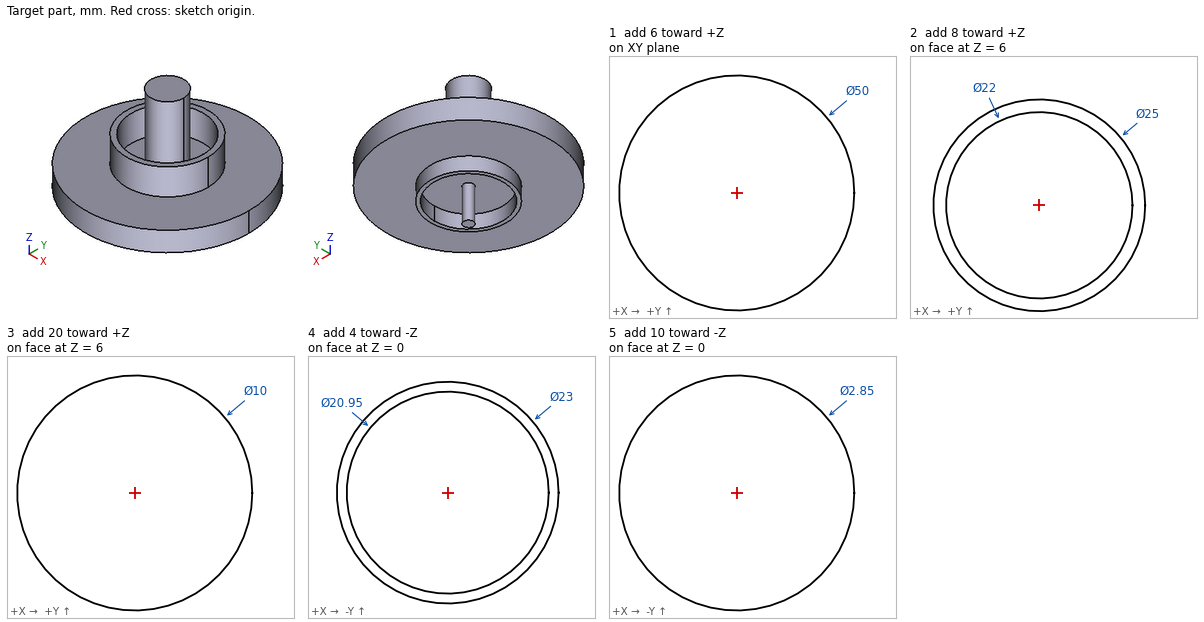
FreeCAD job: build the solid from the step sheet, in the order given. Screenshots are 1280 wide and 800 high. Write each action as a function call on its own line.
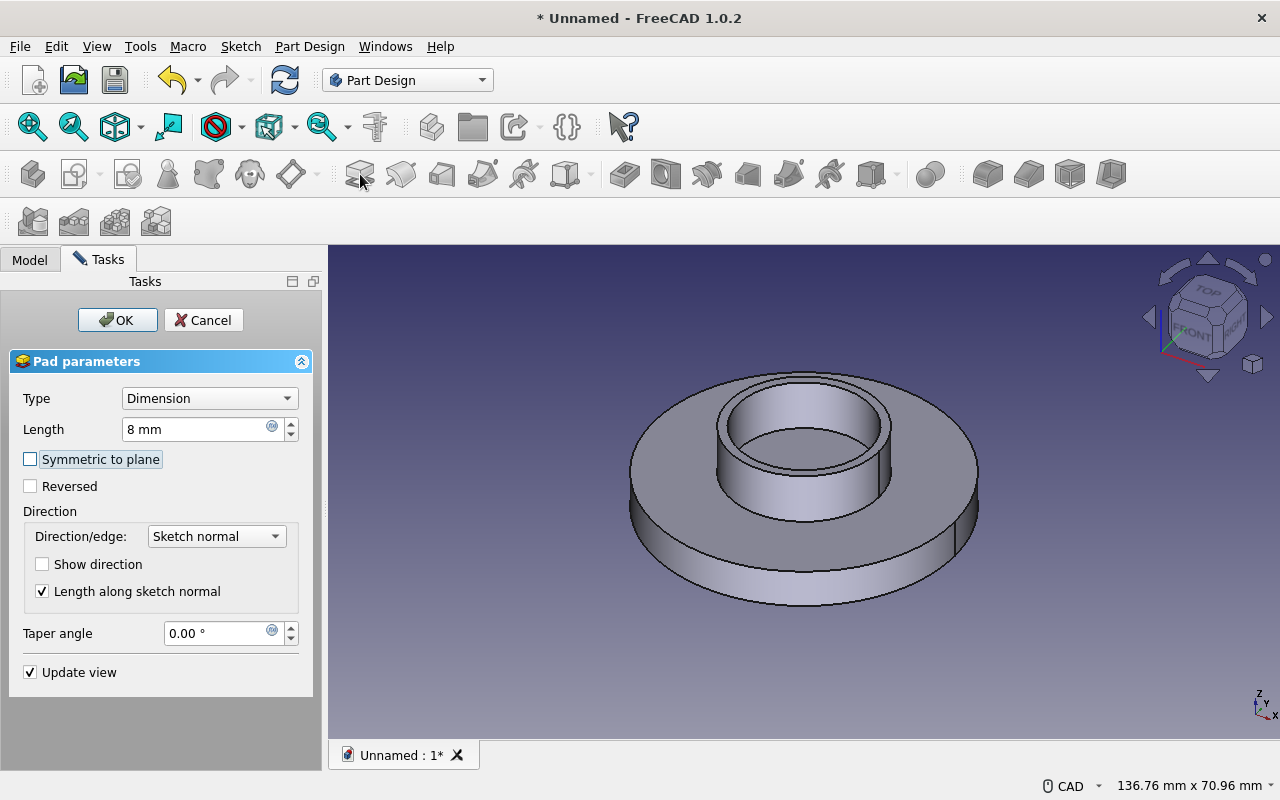
click(118, 320)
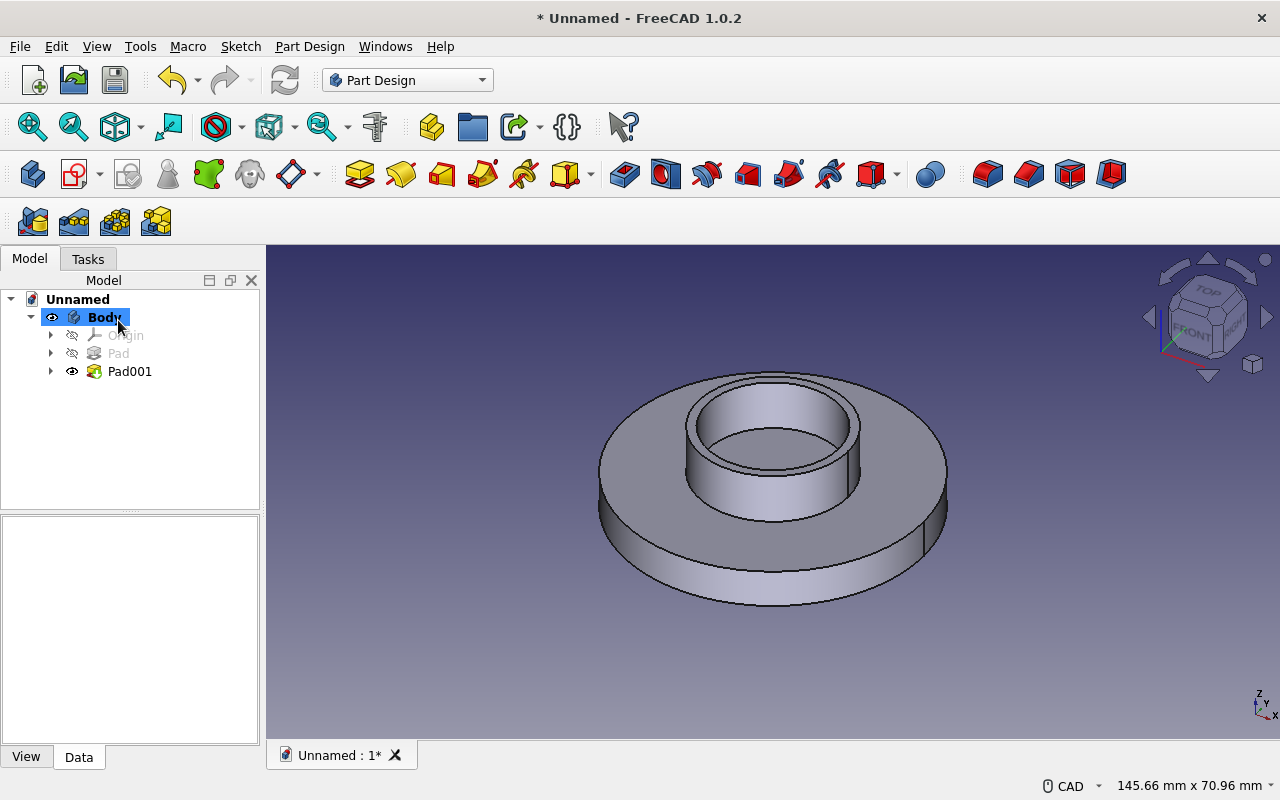
click(809, 549)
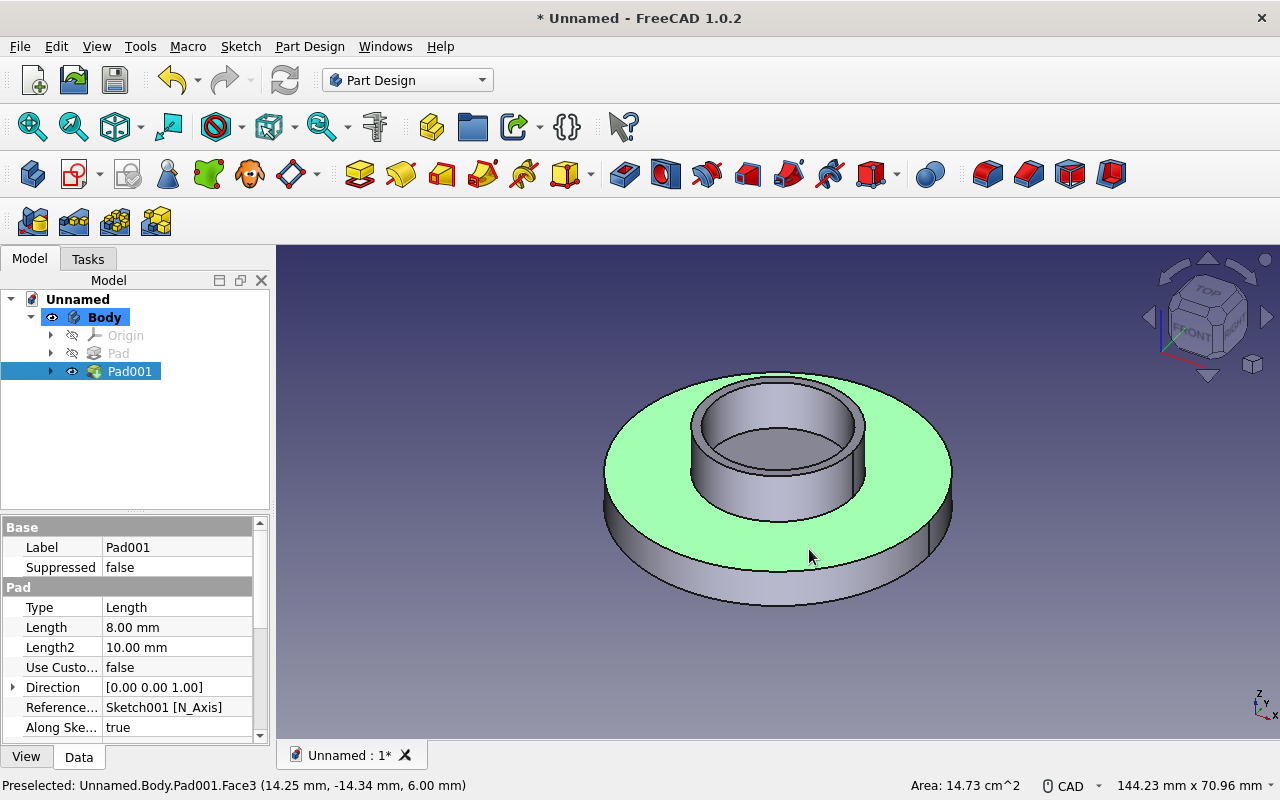
click(74, 174)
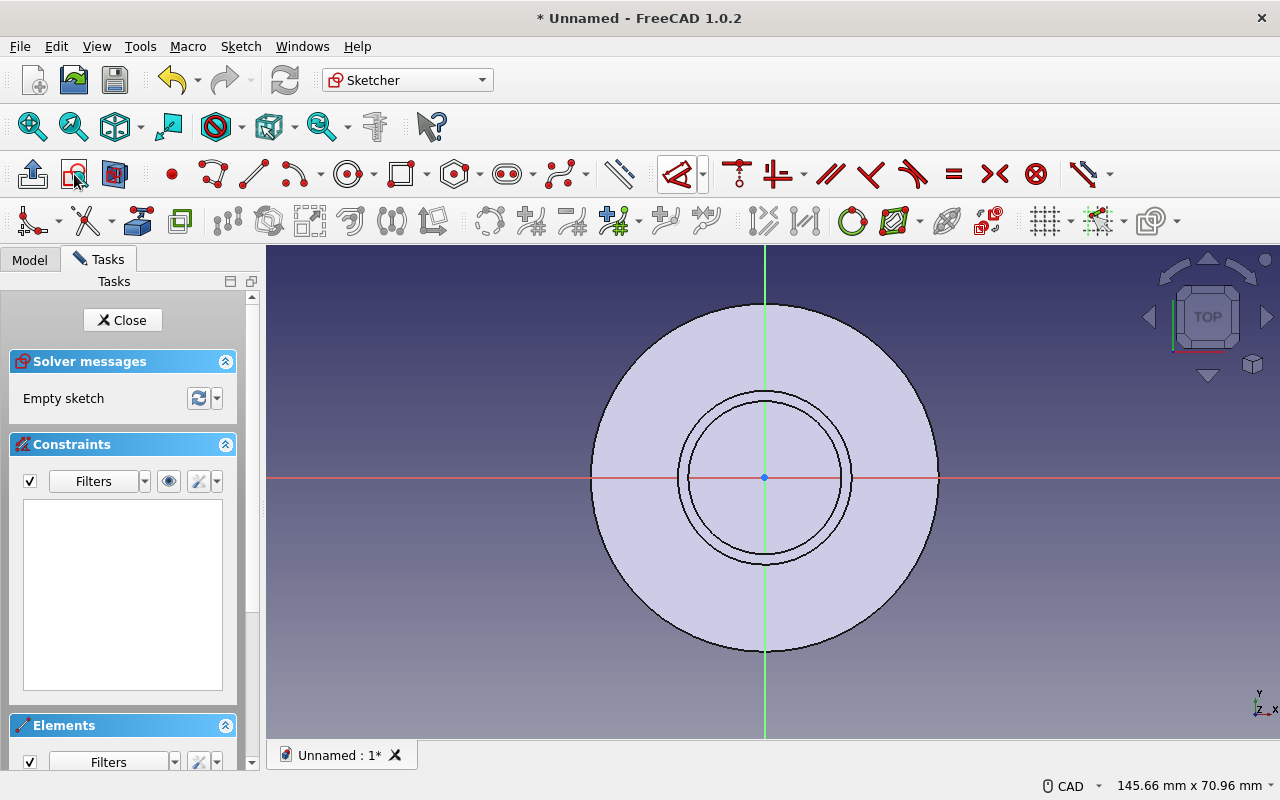
scroll(785, 473, up, 7)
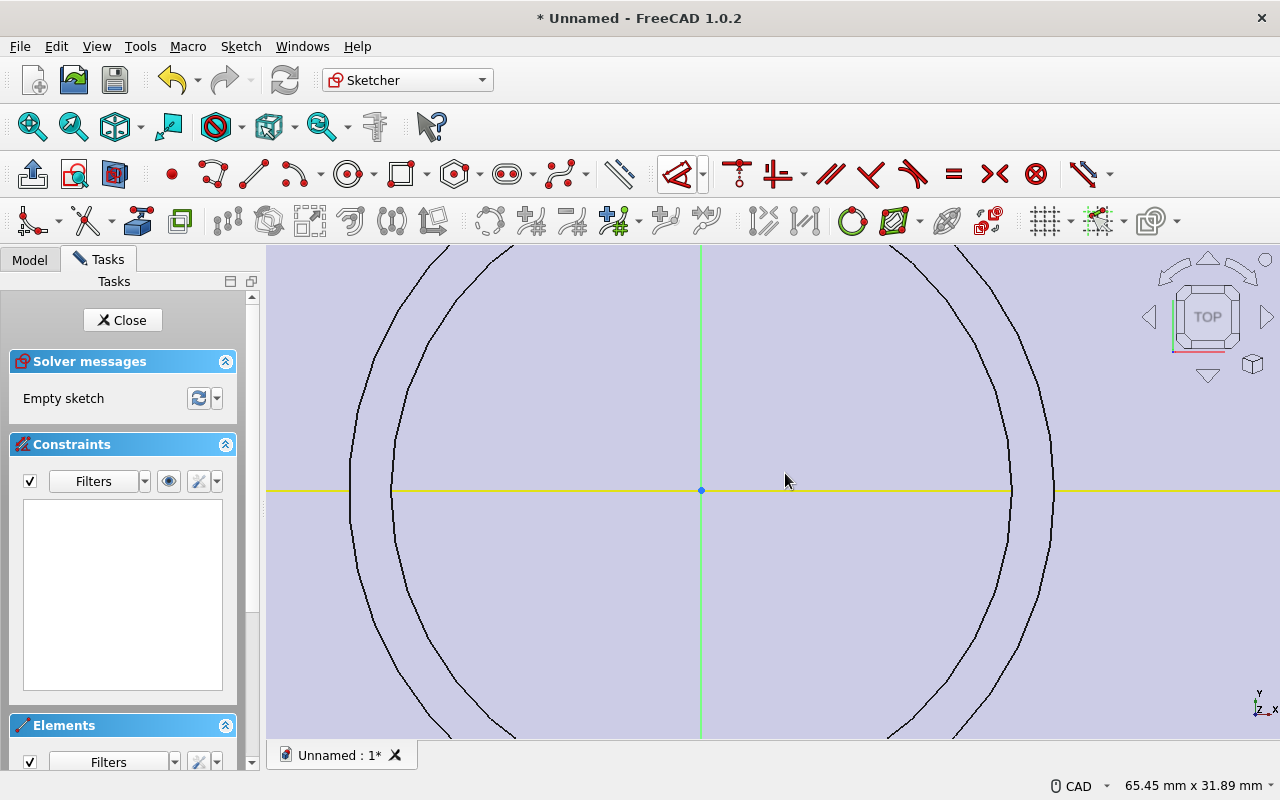
click(348, 174)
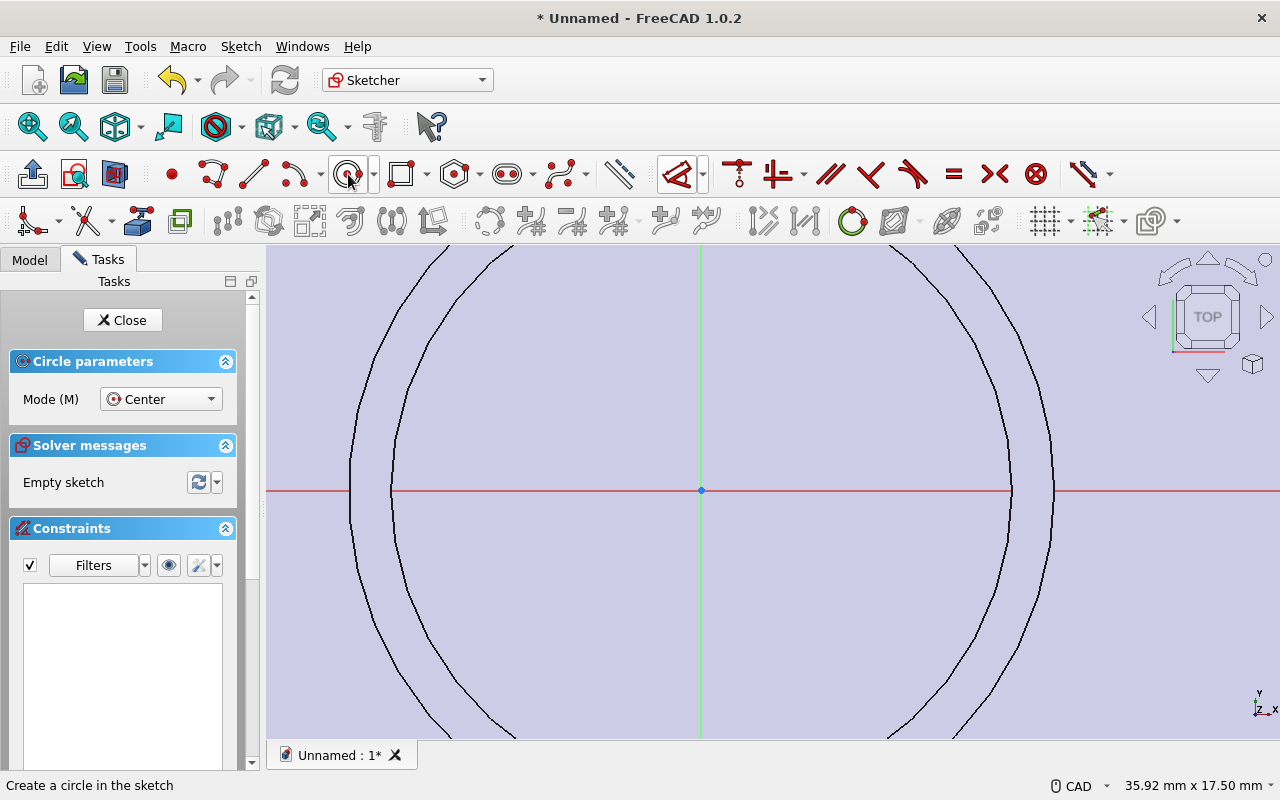
click(701, 491)
click(801, 391)
key(Escape)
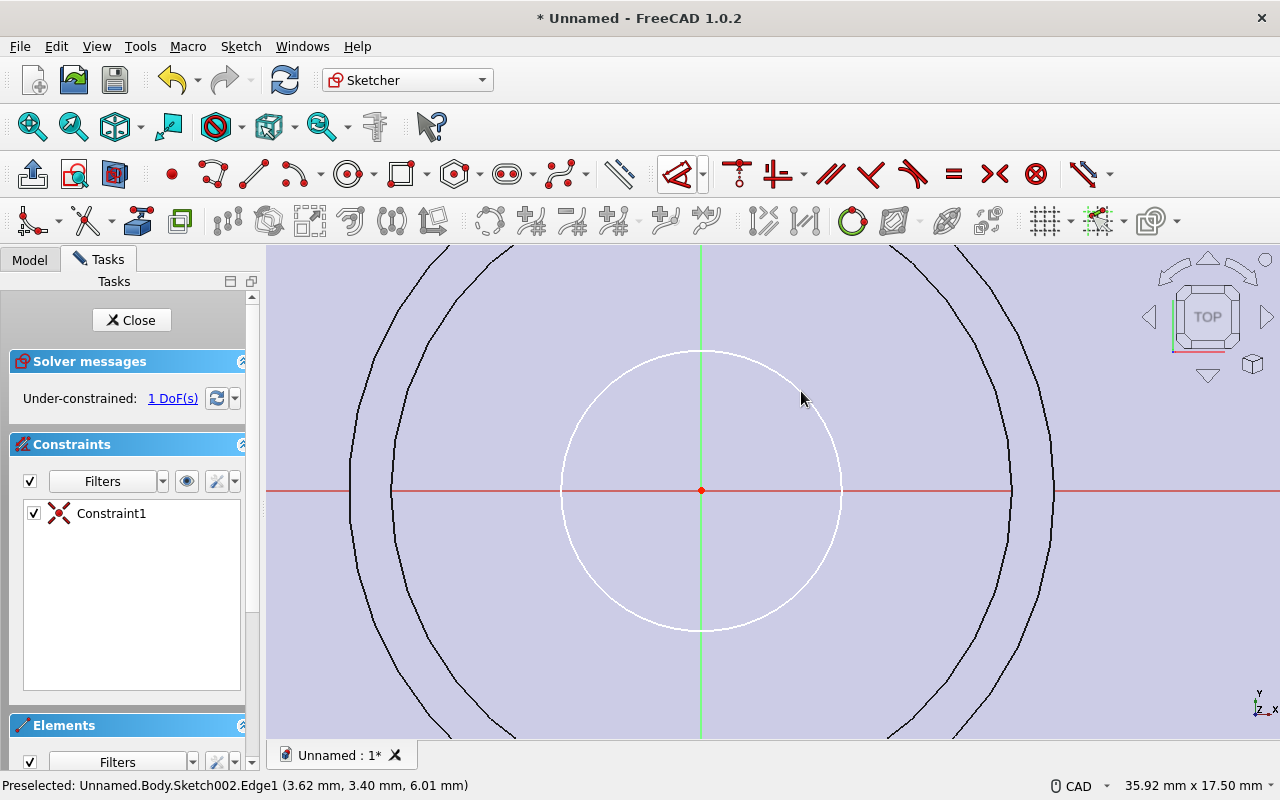
click(800, 391)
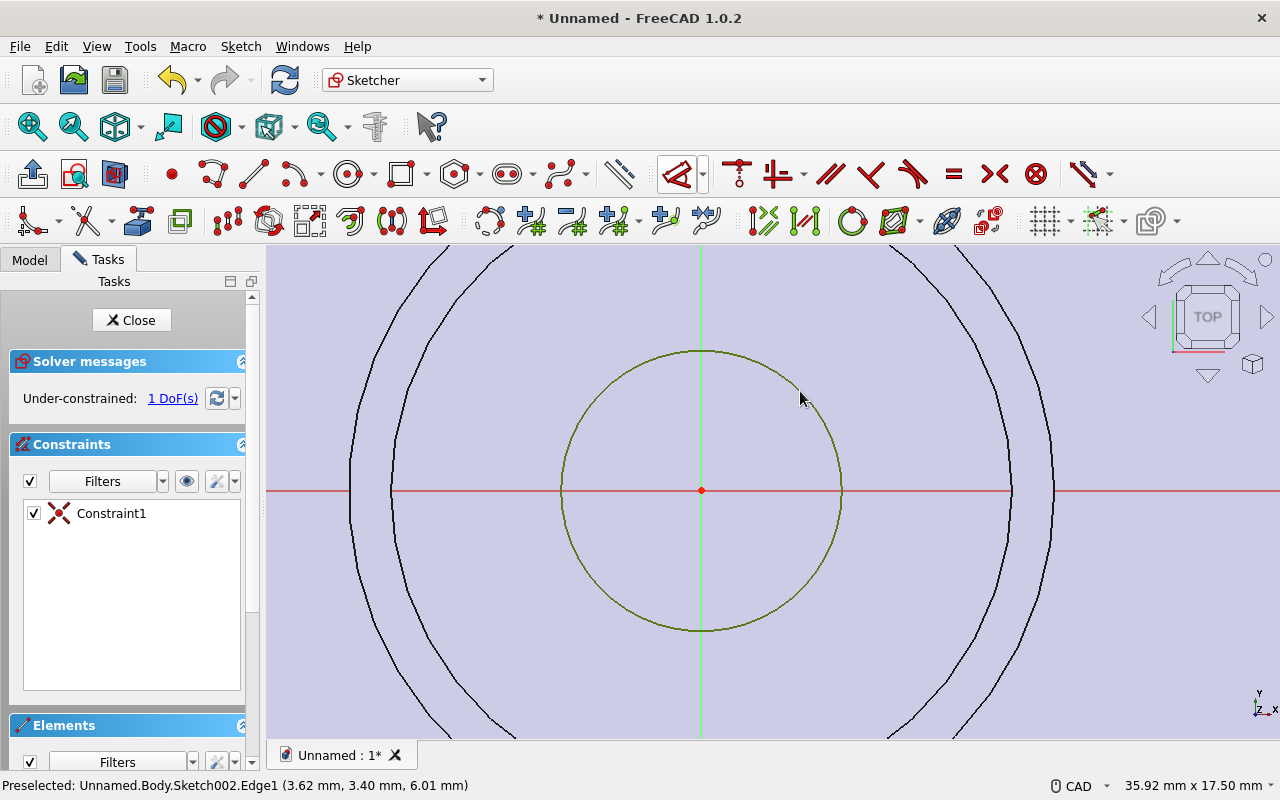
click(702, 174)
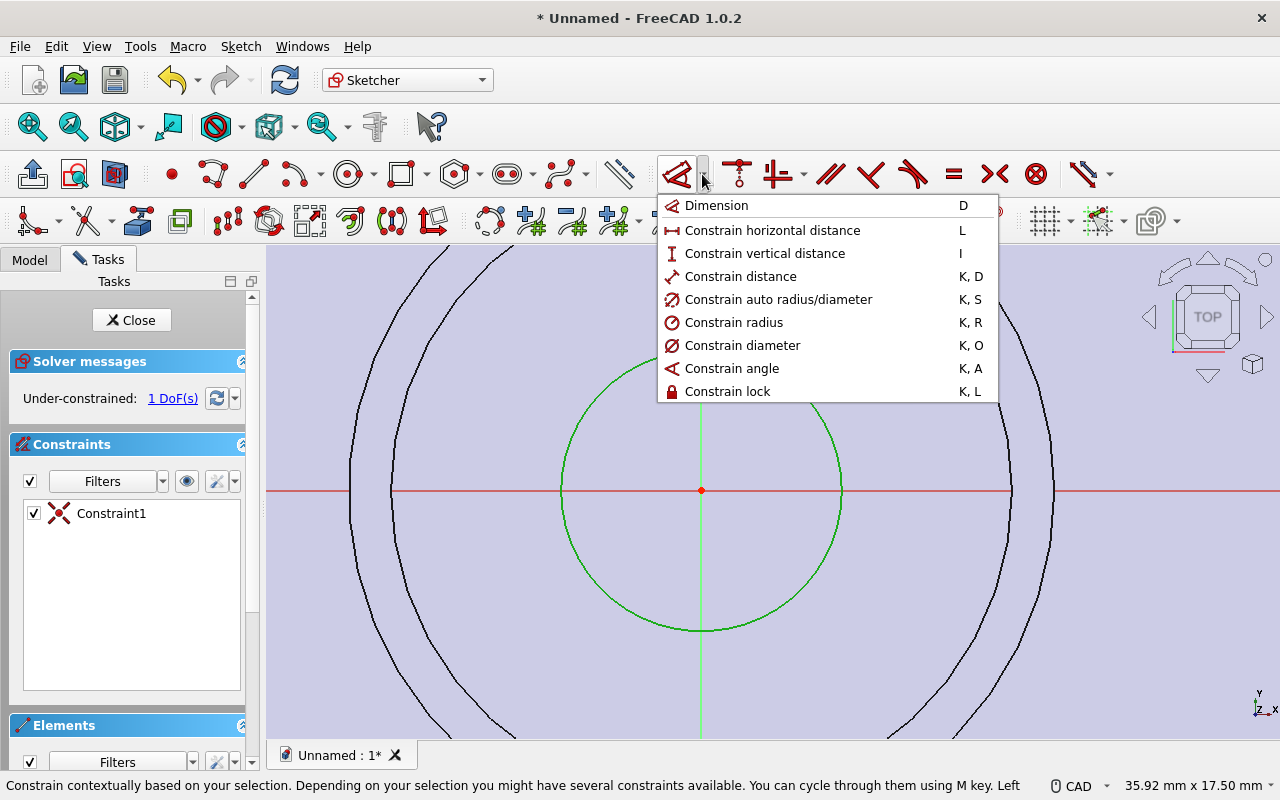
click(828, 346)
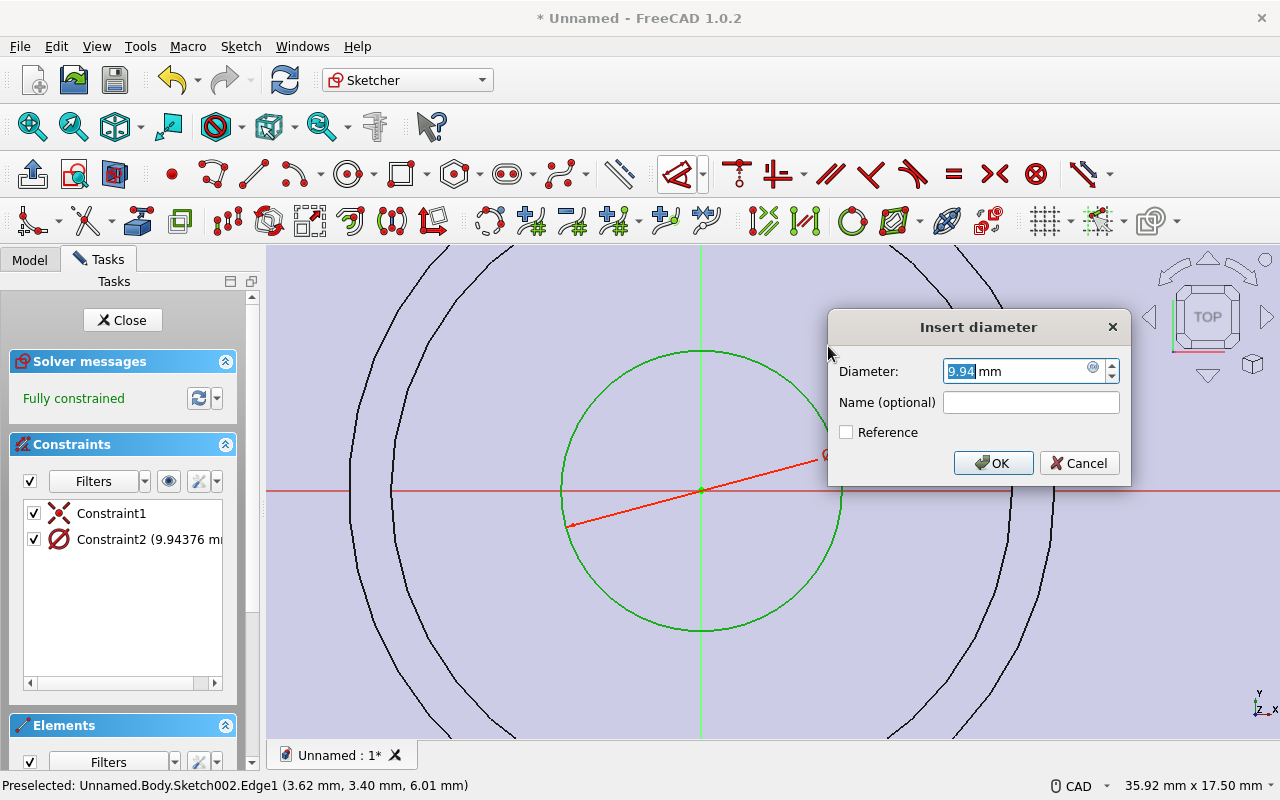
text(10)
key(Return)